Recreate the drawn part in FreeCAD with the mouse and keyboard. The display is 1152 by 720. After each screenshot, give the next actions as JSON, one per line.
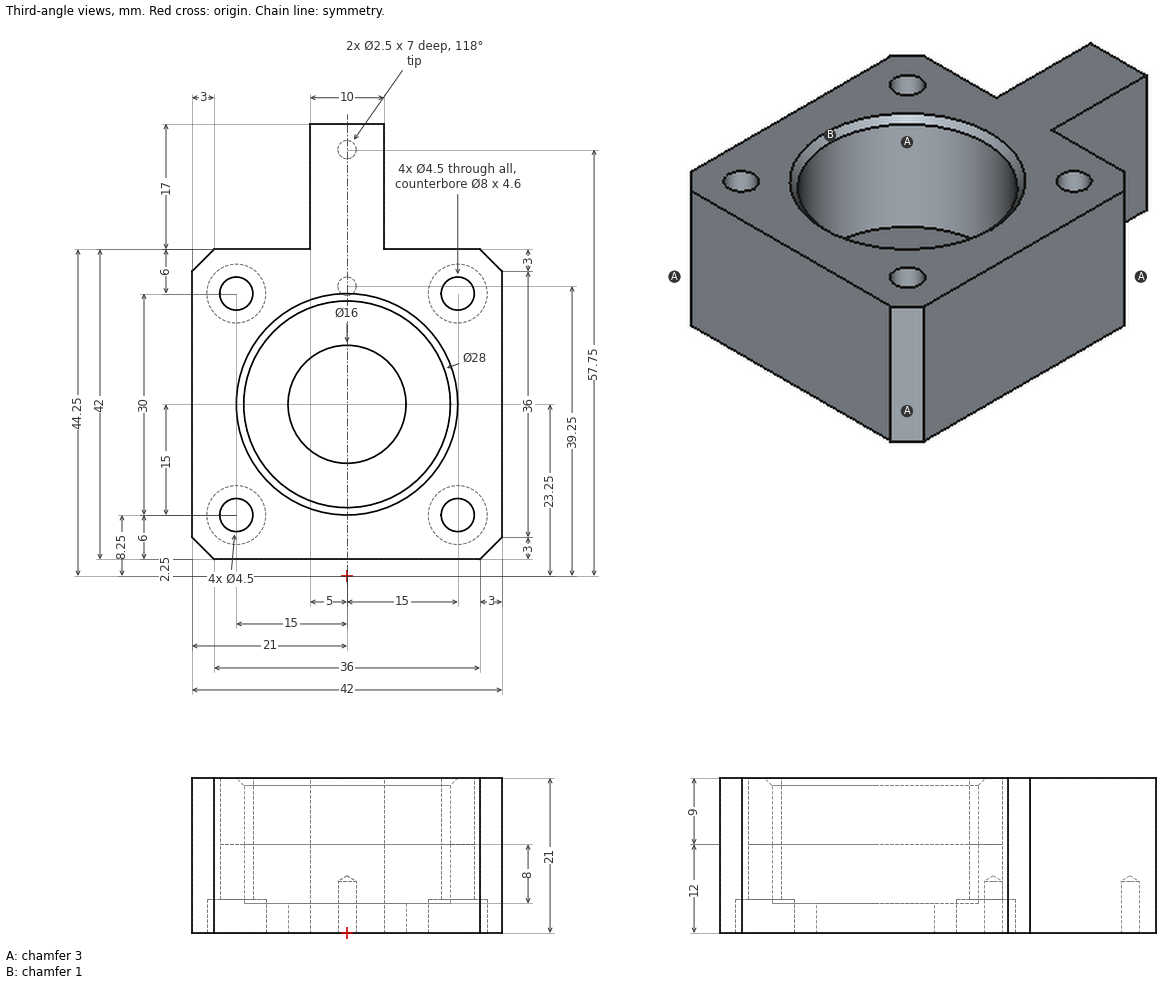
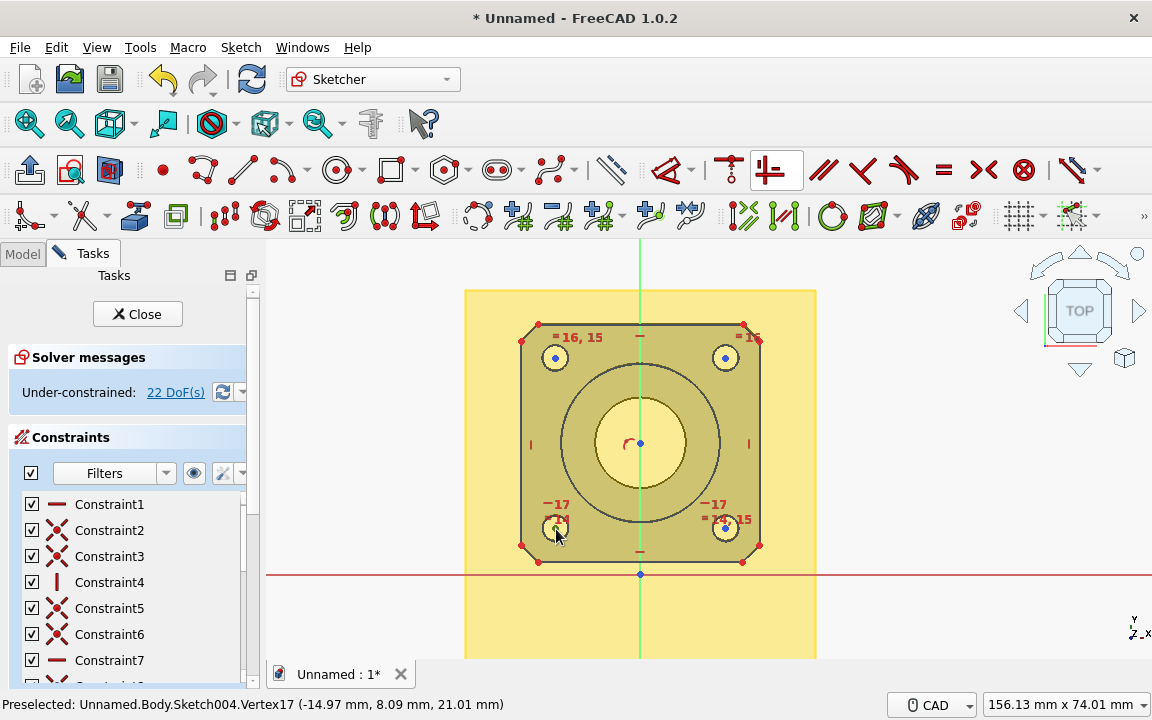
{"action": "left_click", "coordinate": [555, 358]}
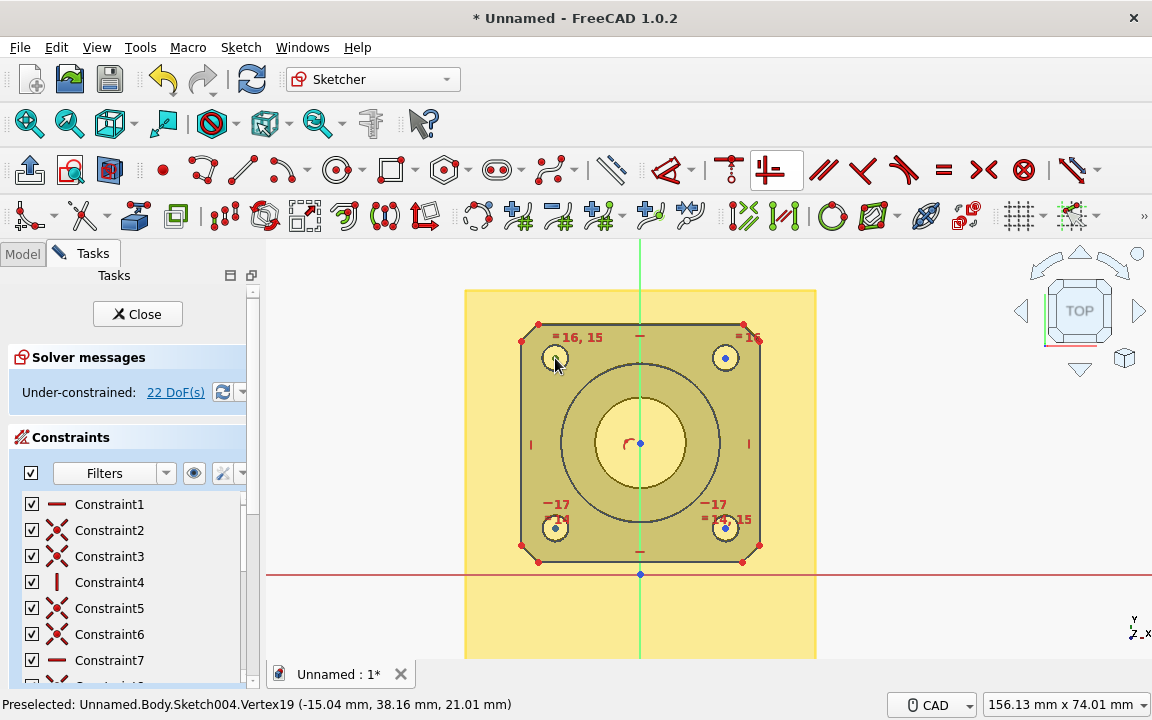
{"action": "left_click", "coordinate": [798, 170]}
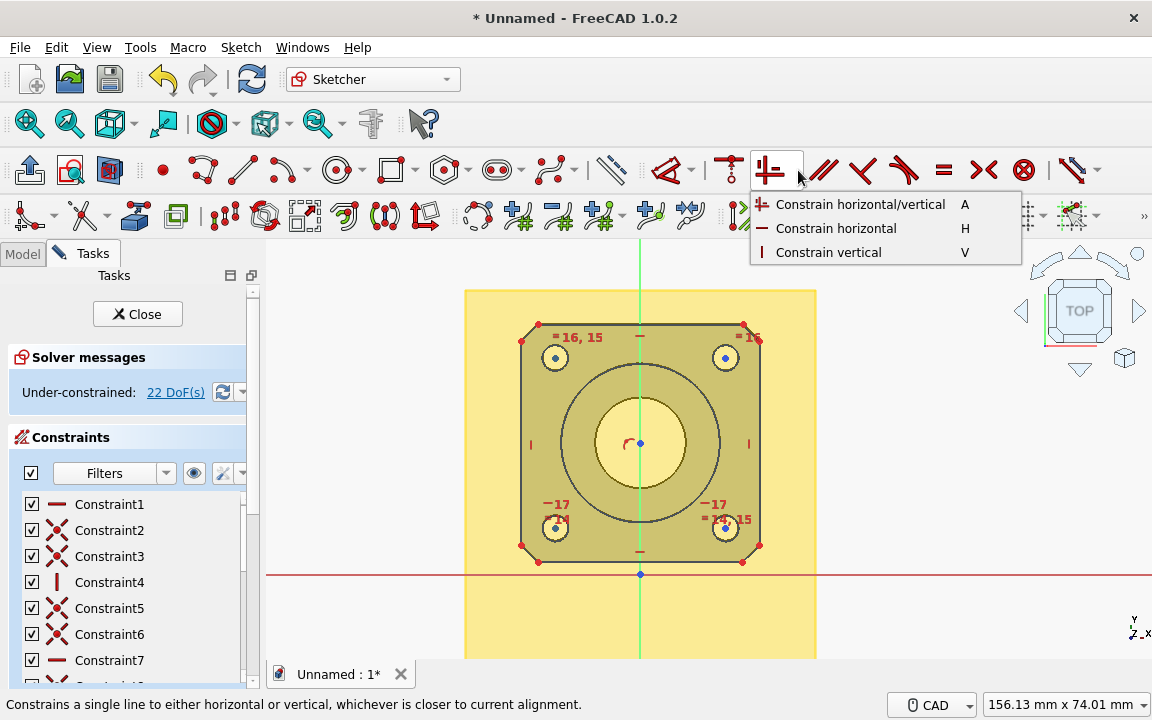
{"action": "left_click", "coordinate": [886, 252]}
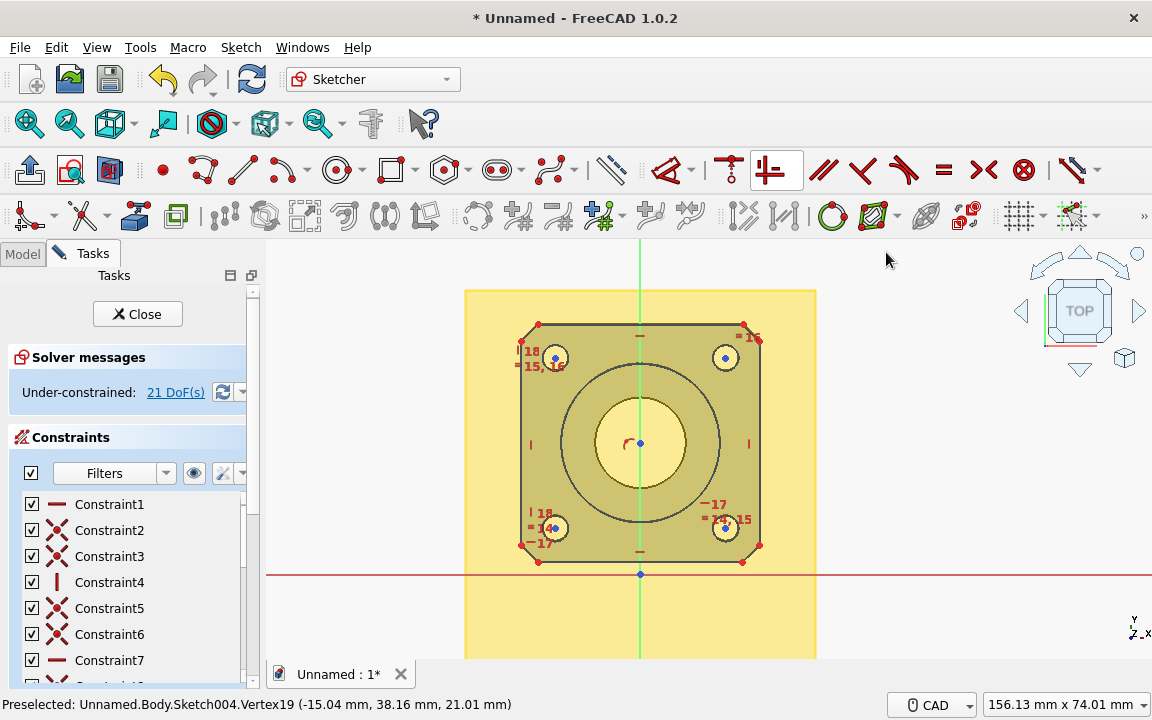
{"action": "left_click", "coordinate": [726, 529]}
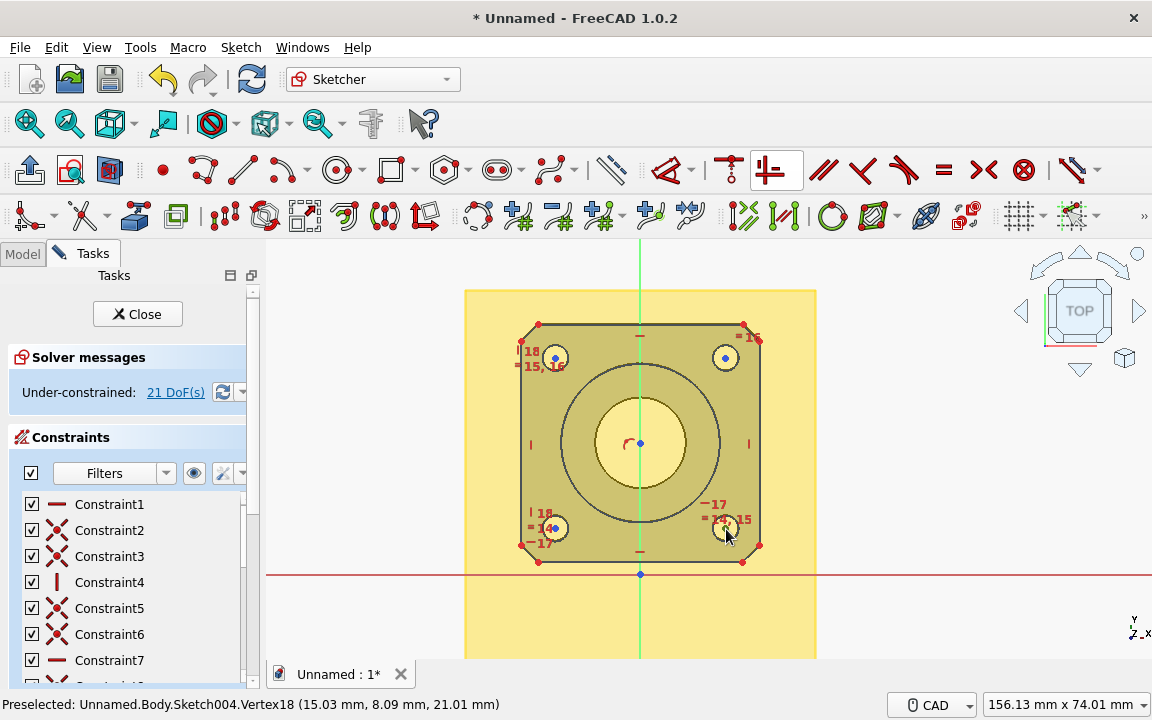
{"action": "left_click", "coordinate": [726, 358]}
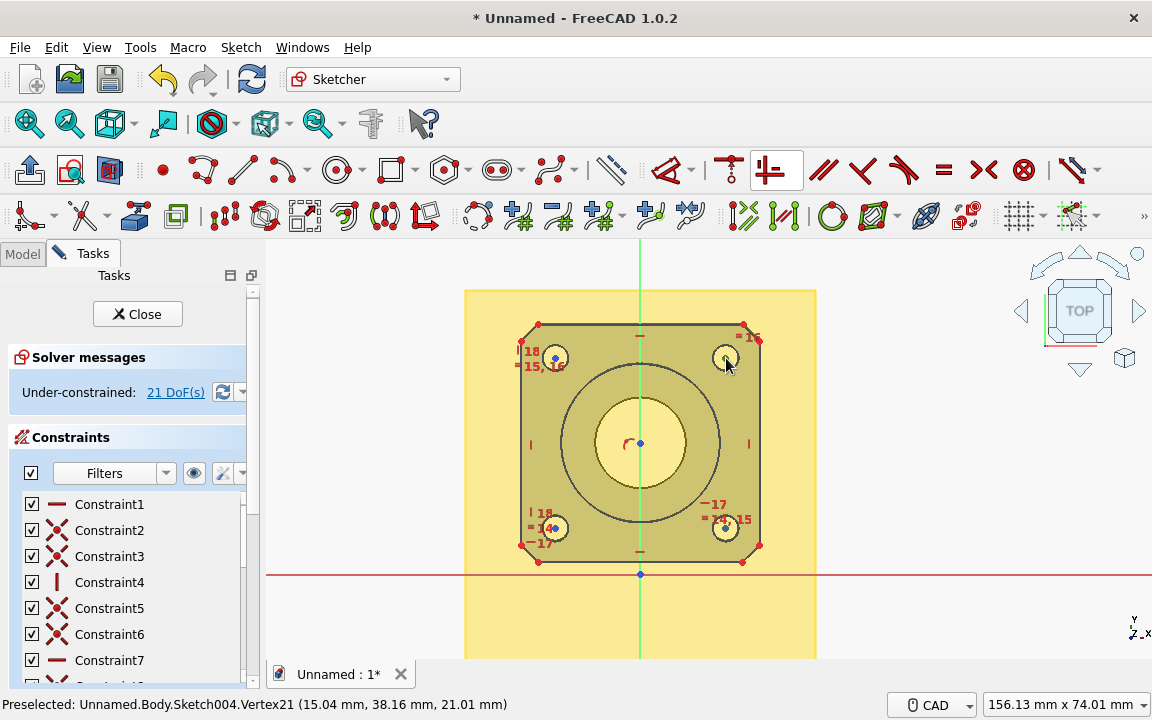
{"action": "left_click", "coordinate": [798, 170]}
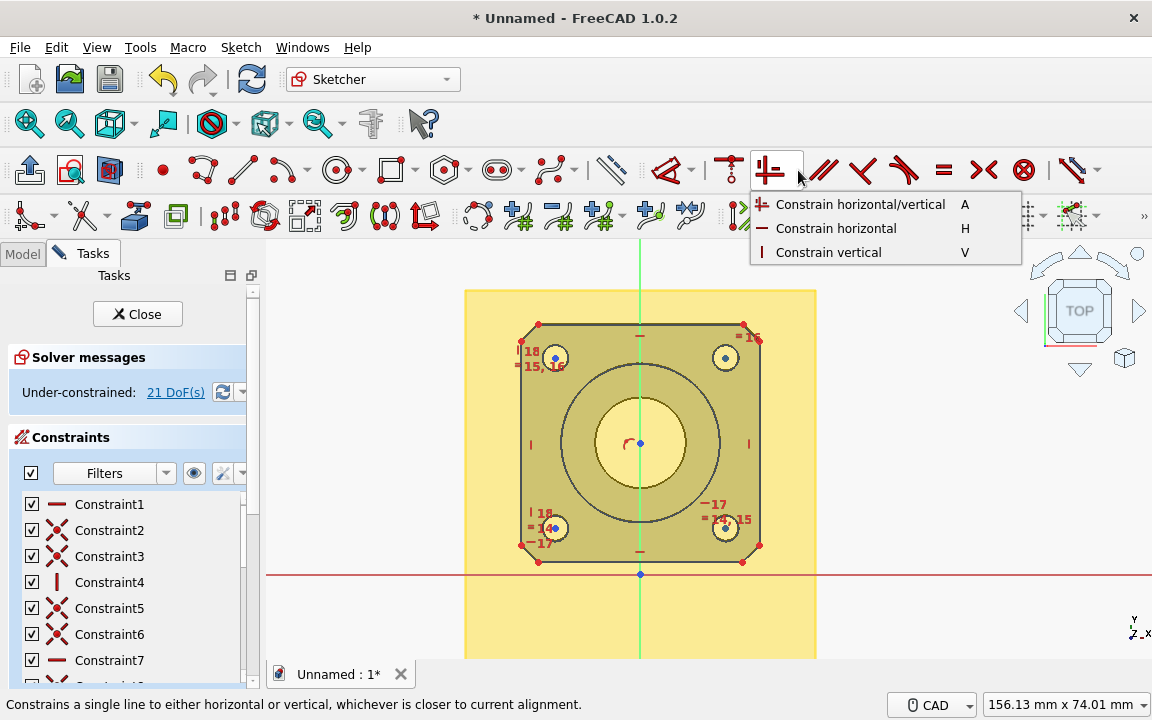
{"action": "left_click", "coordinate": [886, 252]}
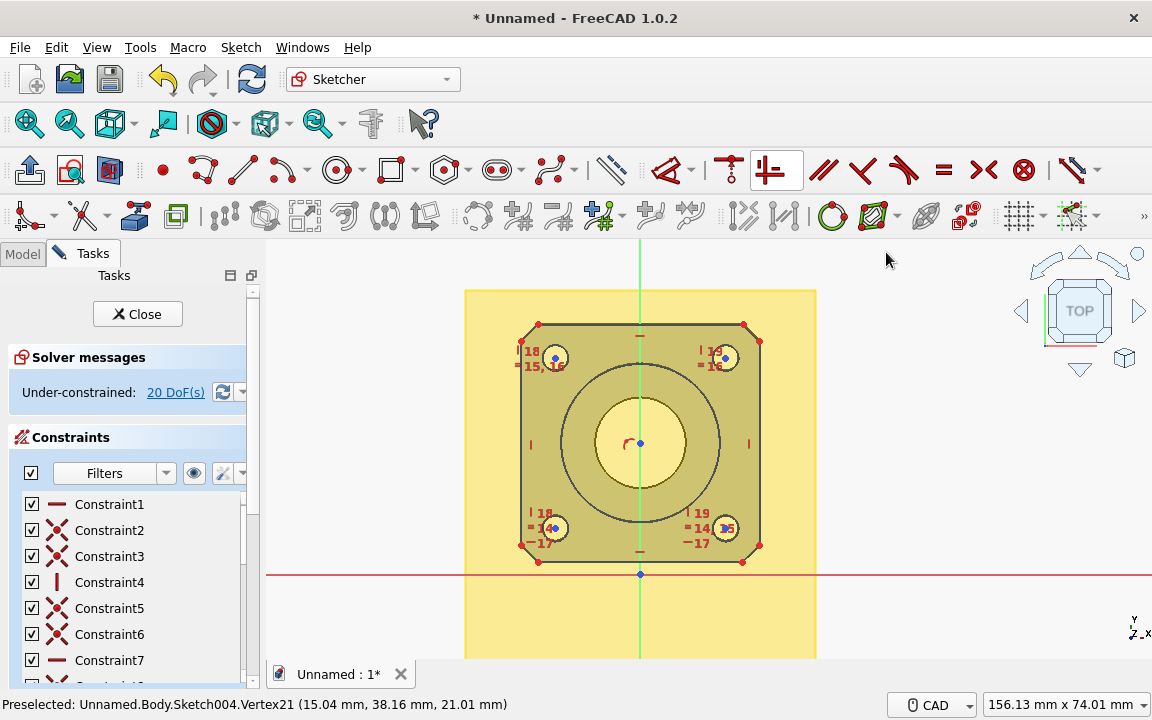
{"action": "scroll", "coordinate": [556, 358], "scroll_direction": "up", "scroll_amount": 4}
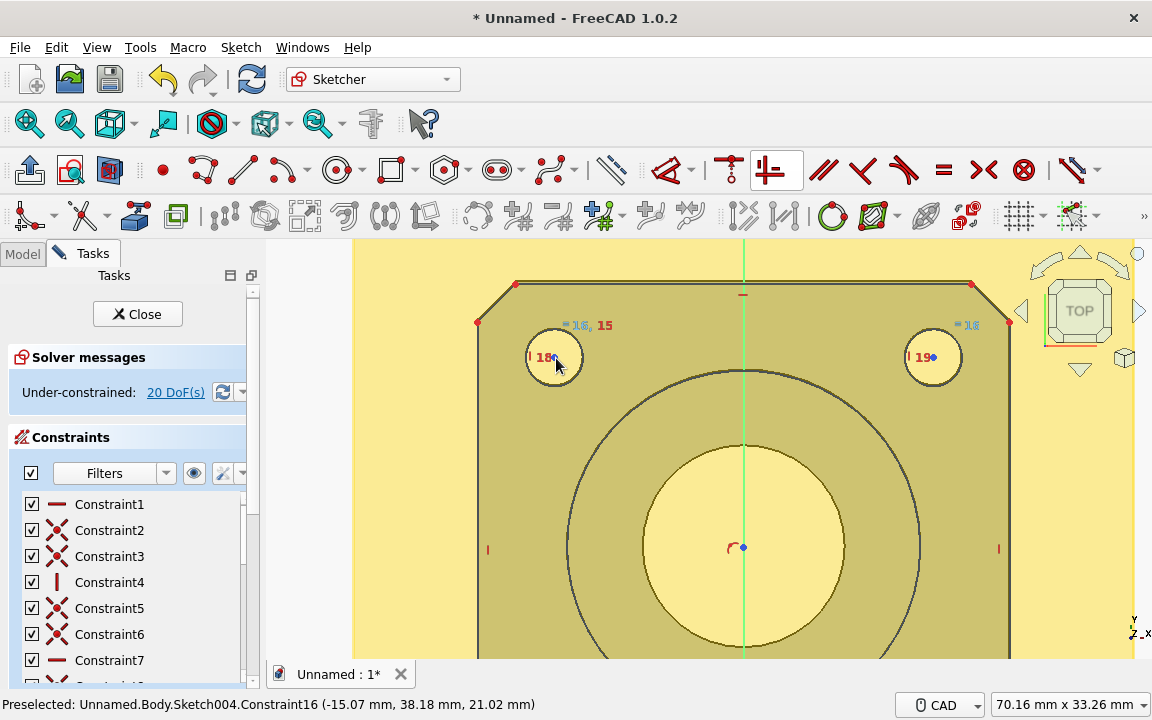
{"action": "left_click", "coordinate": [555, 358]}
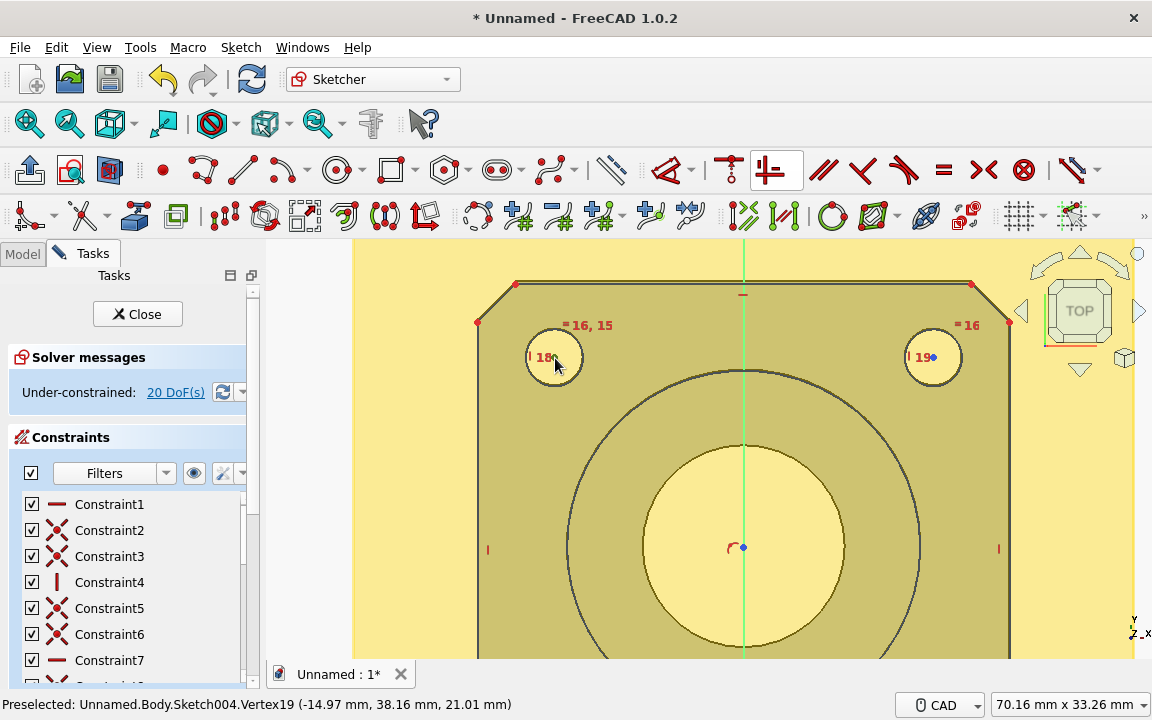
{"action": "left_click", "coordinate": [933, 358]}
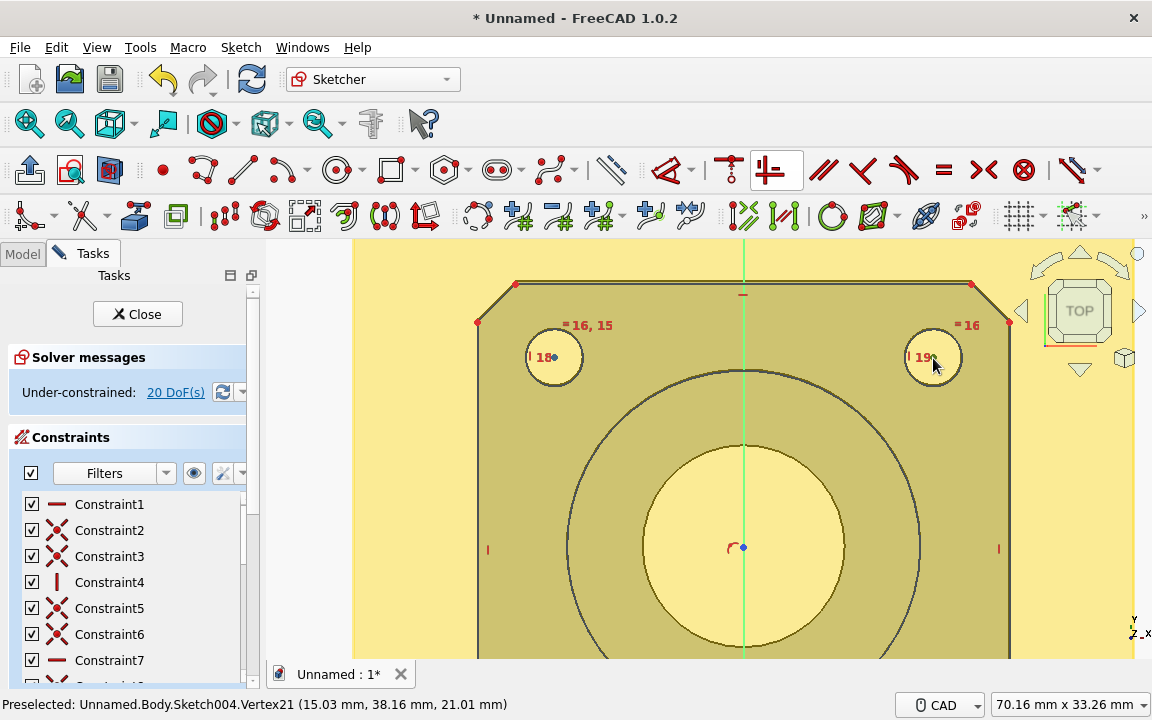
{"action": "left_click", "coordinate": [744, 605]}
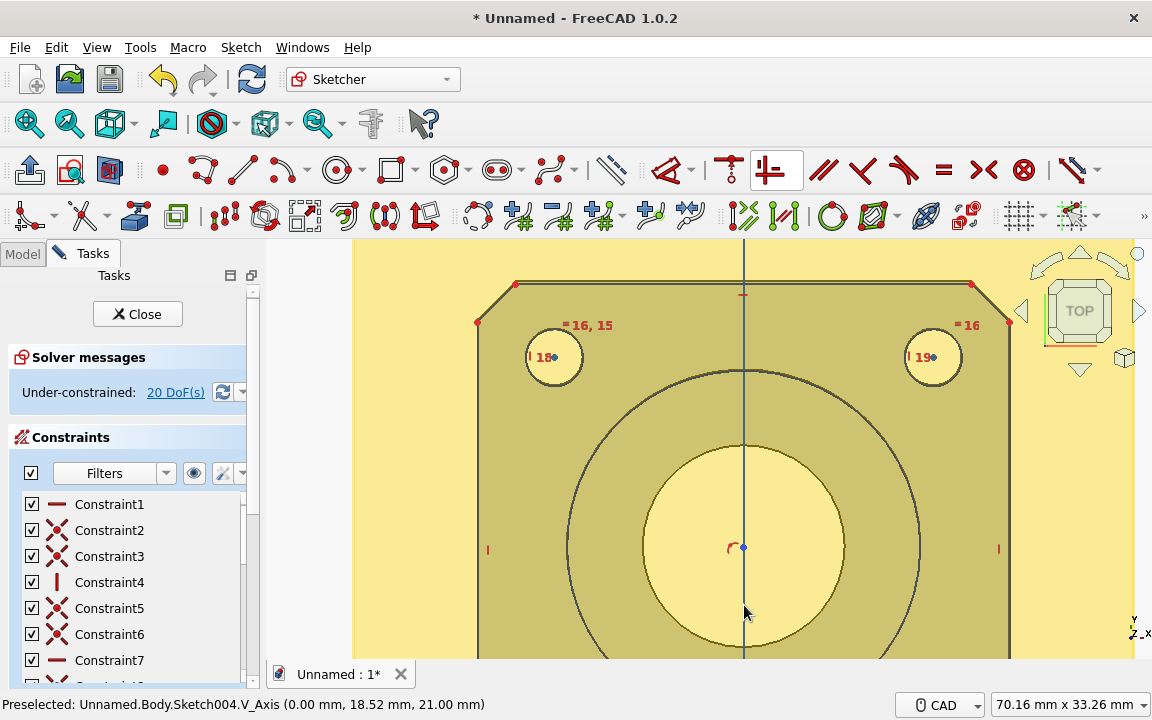
{"action": "left_click", "coordinate": [984, 170]}